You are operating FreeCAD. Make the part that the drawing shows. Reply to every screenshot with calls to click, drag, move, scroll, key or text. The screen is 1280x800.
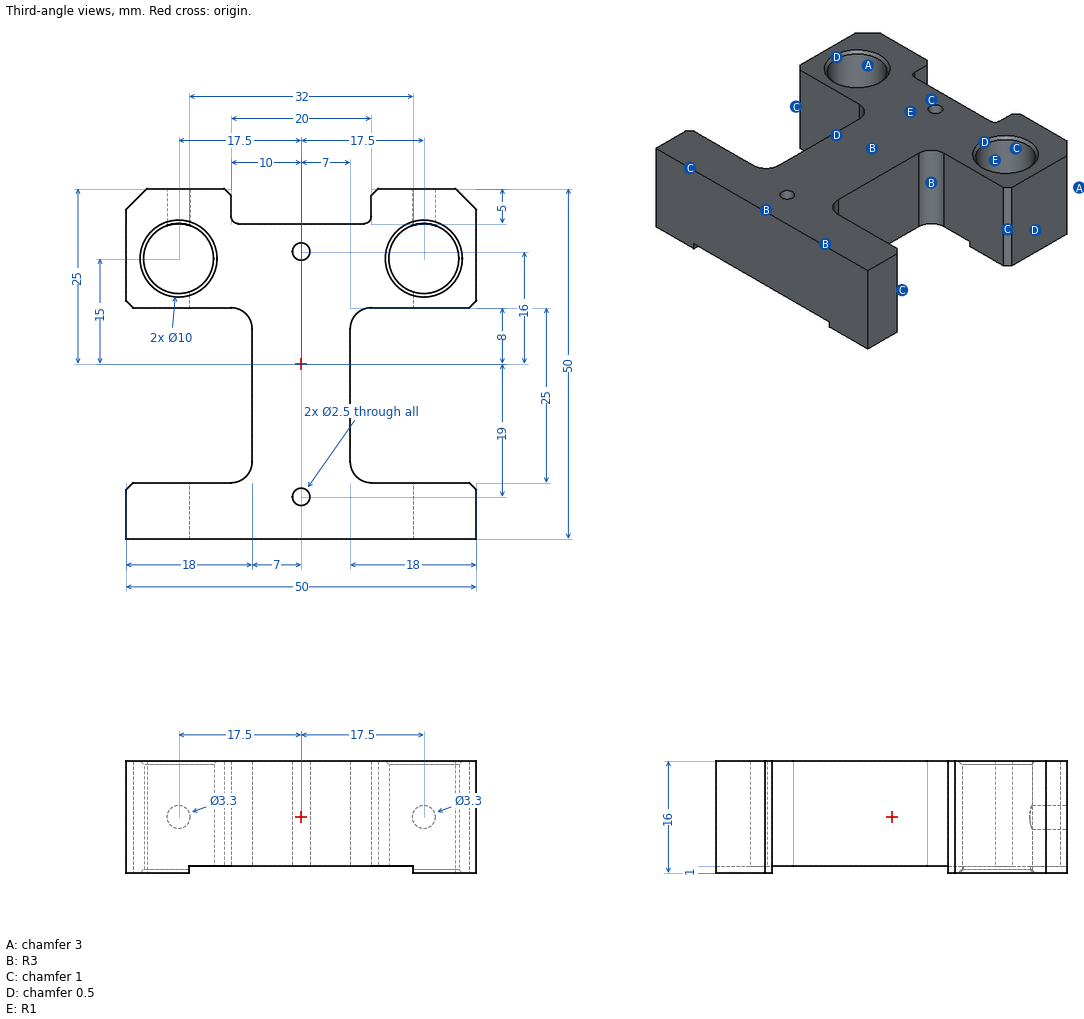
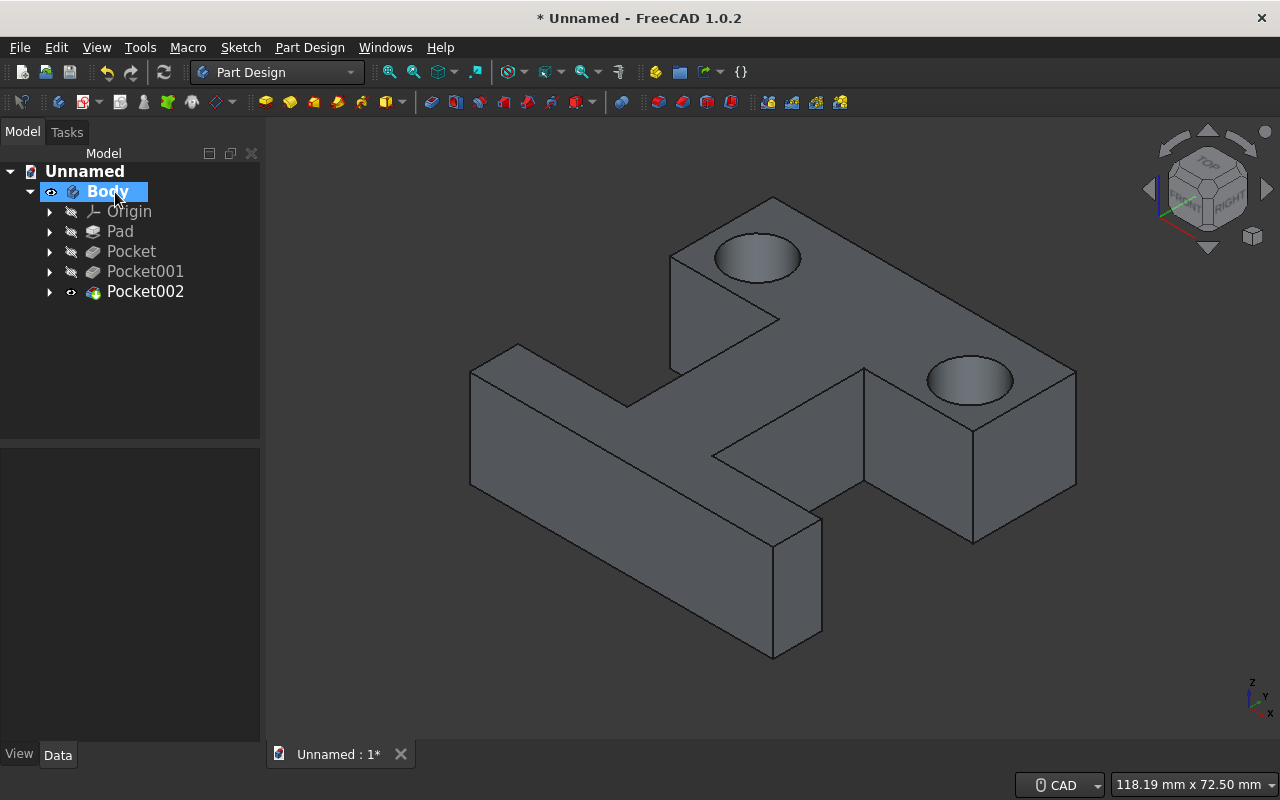
click(860, 321)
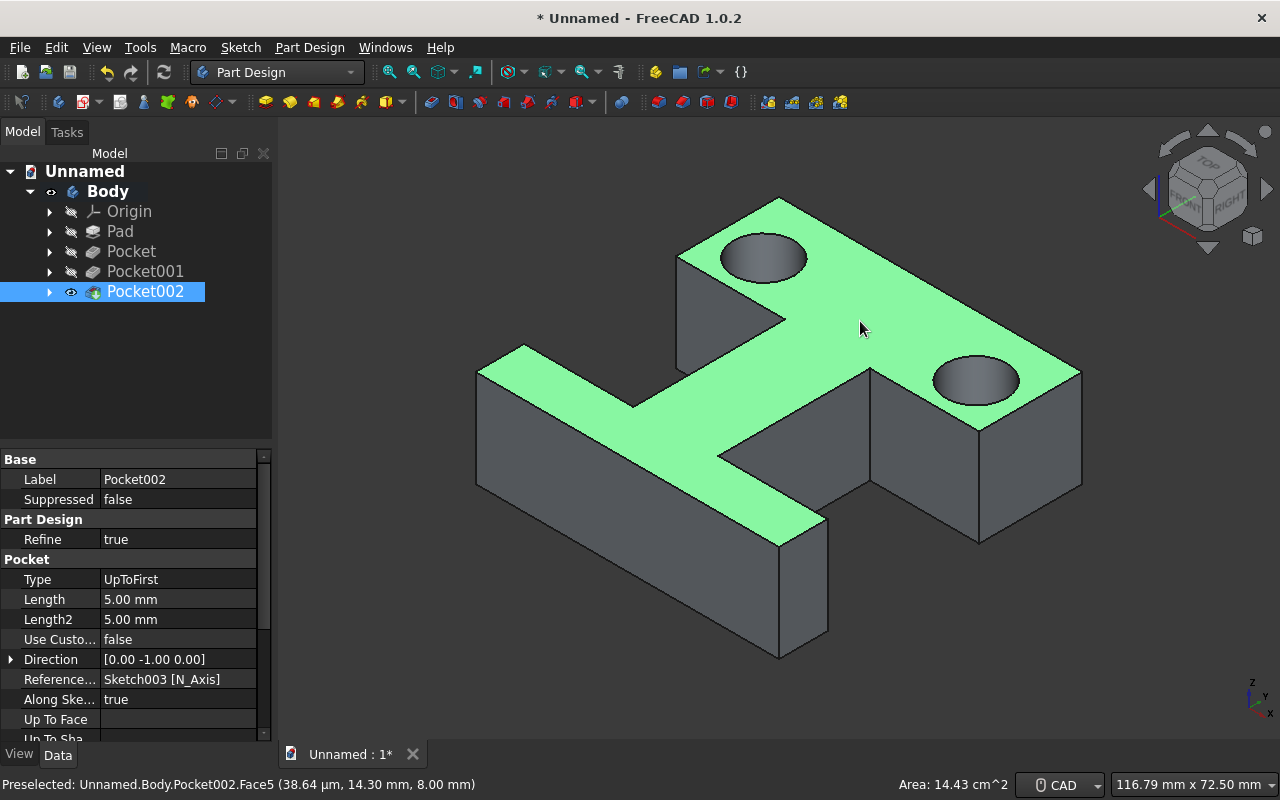
click(84, 102)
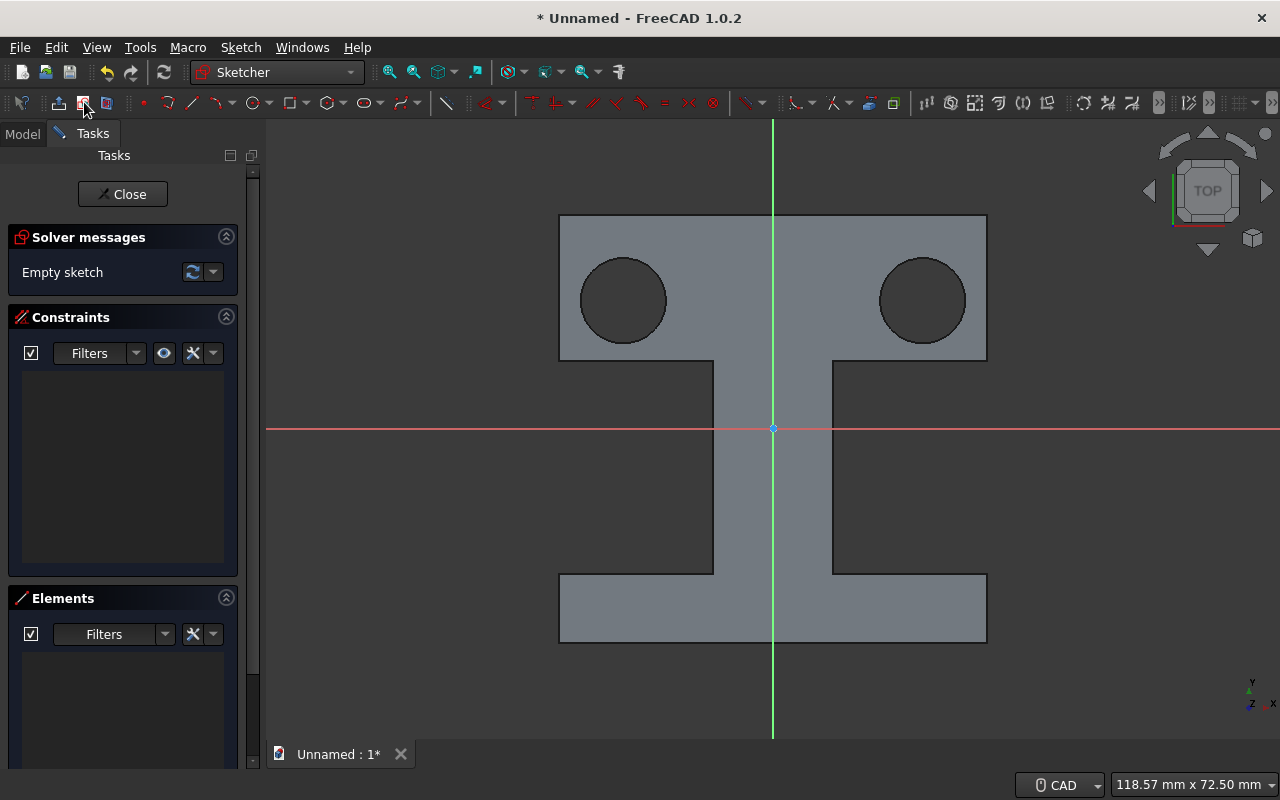
key(g)
key(c)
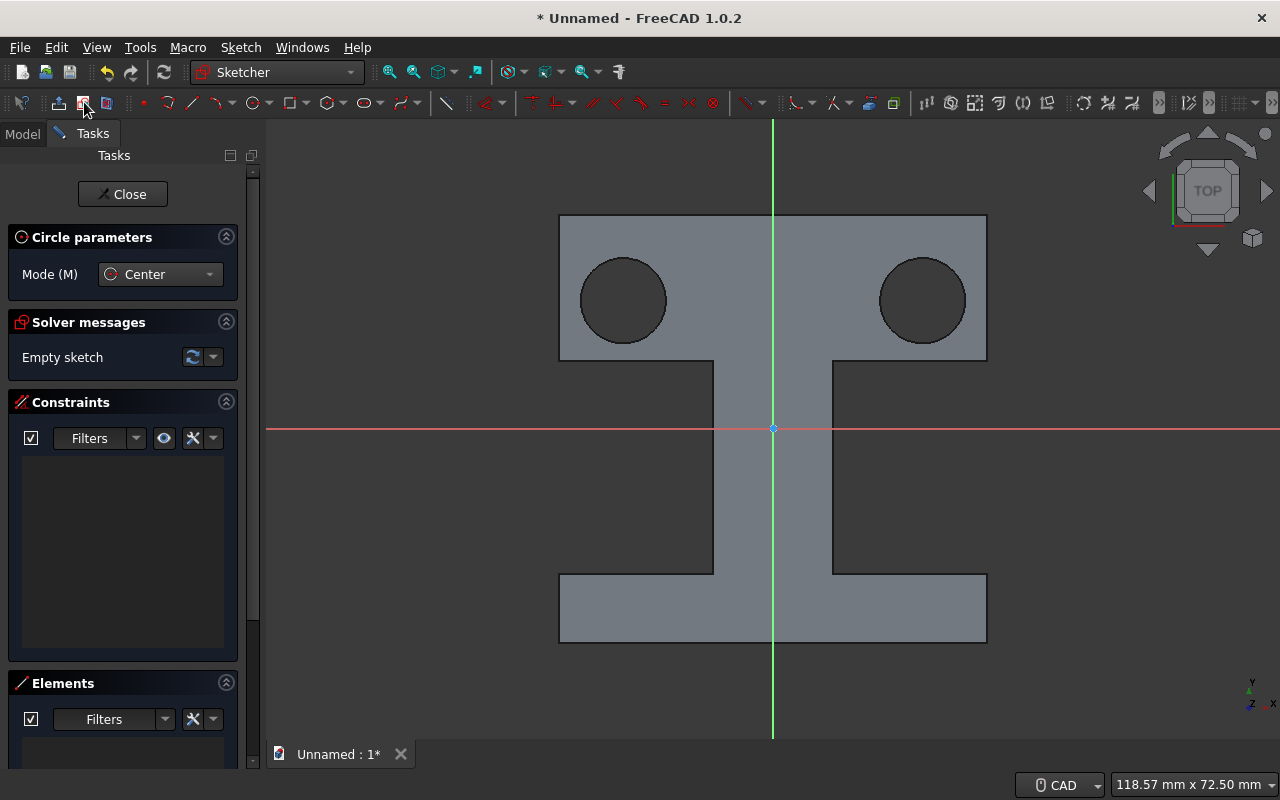
scroll(773, 591, up, 4)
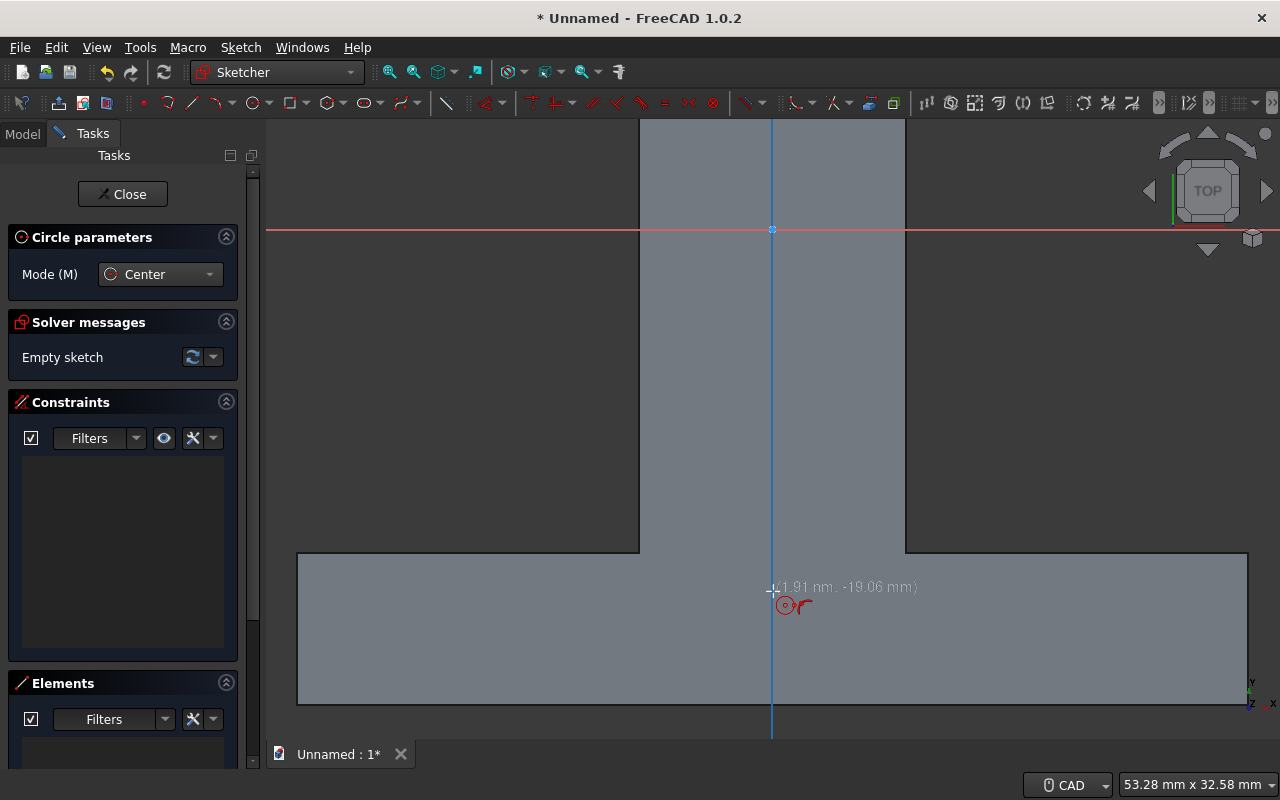
click(772, 591)
move(789, 574)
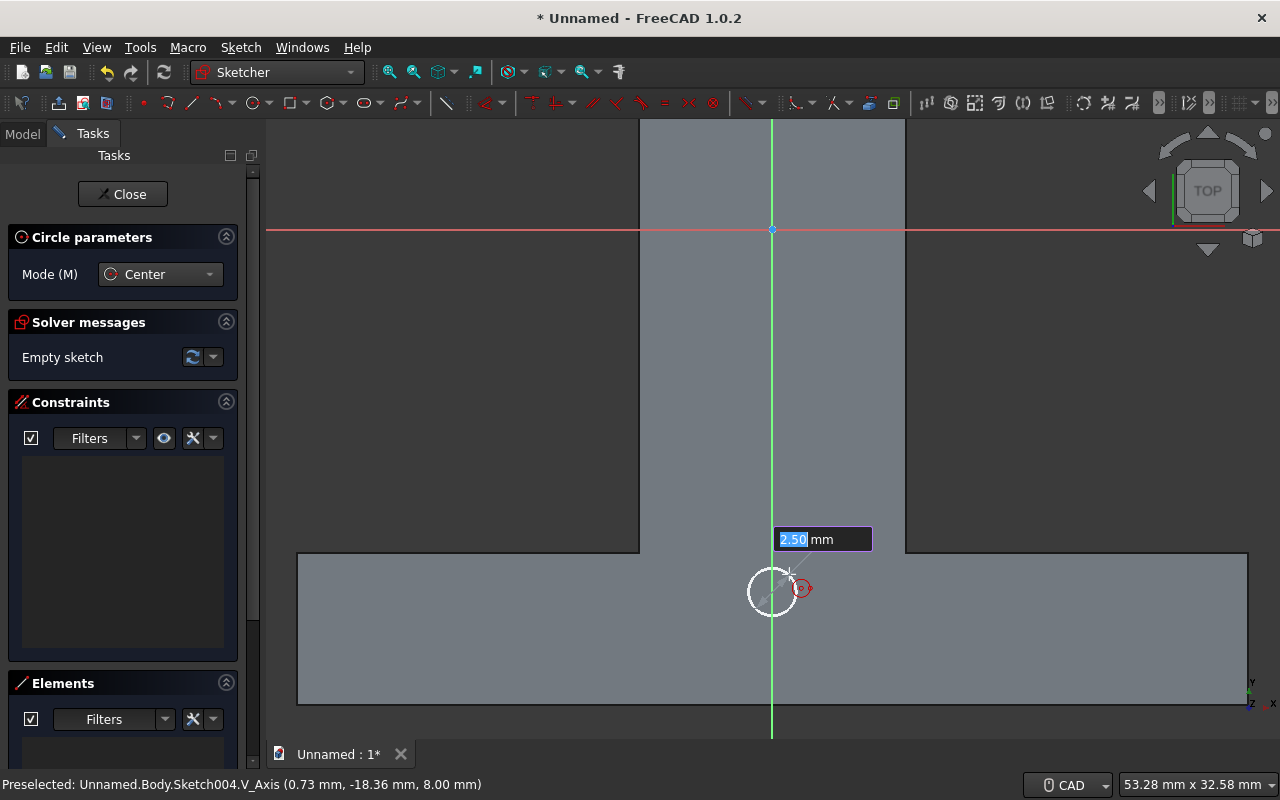
text(2.5)
key(Return)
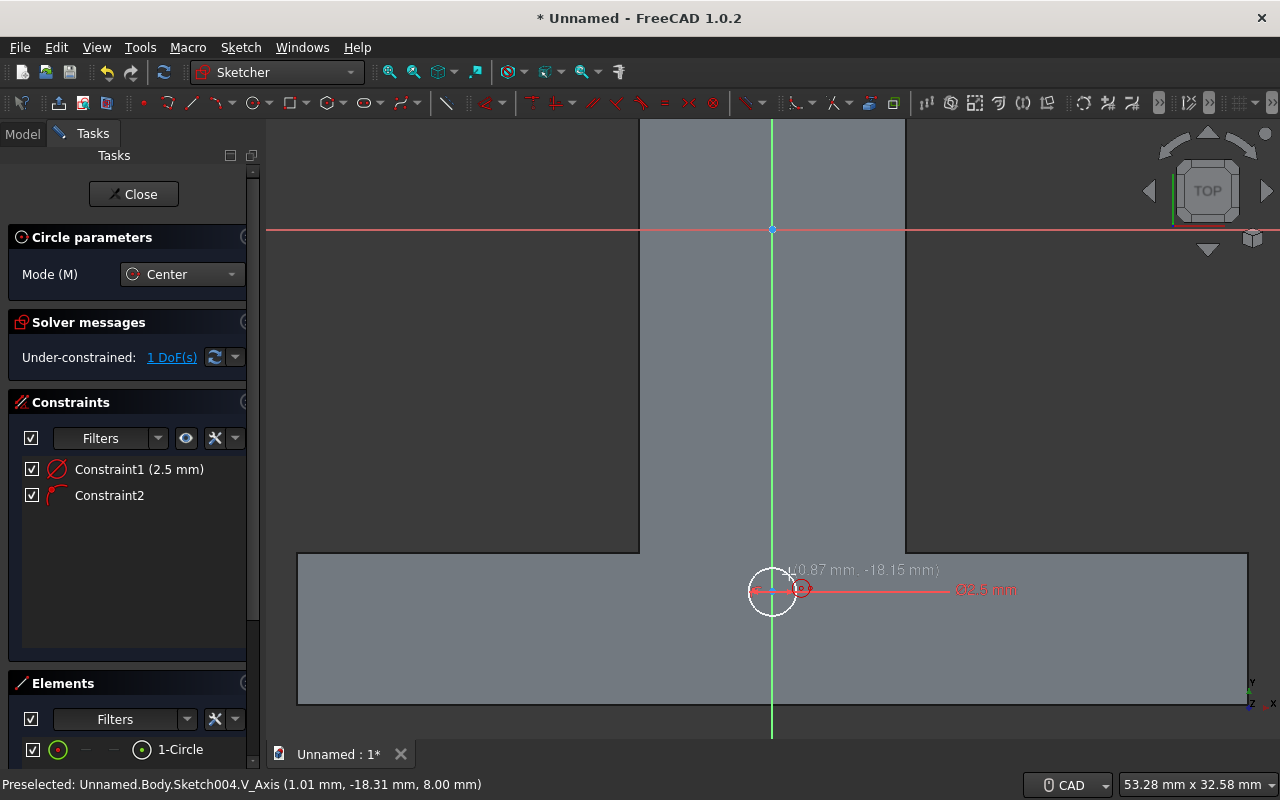
scroll(622, 637, down, 3)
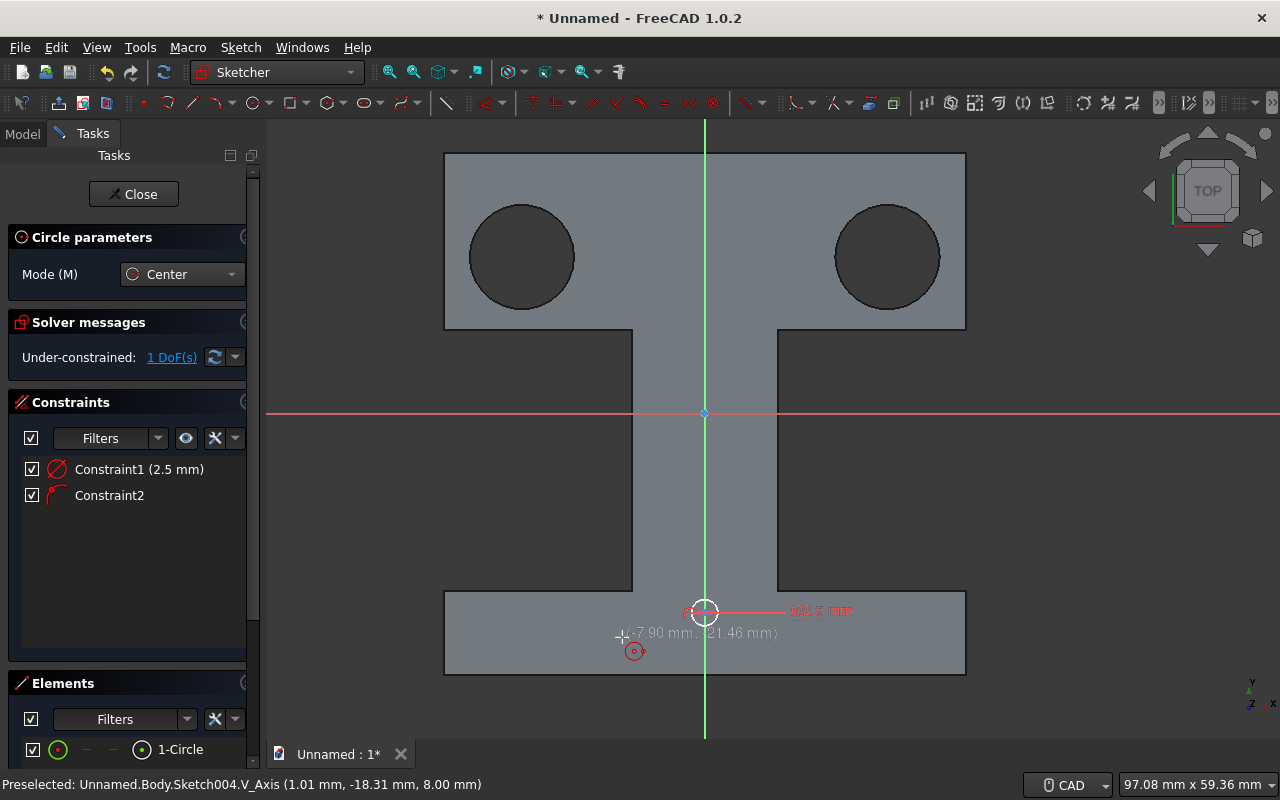
scroll(705, 247, up, 3)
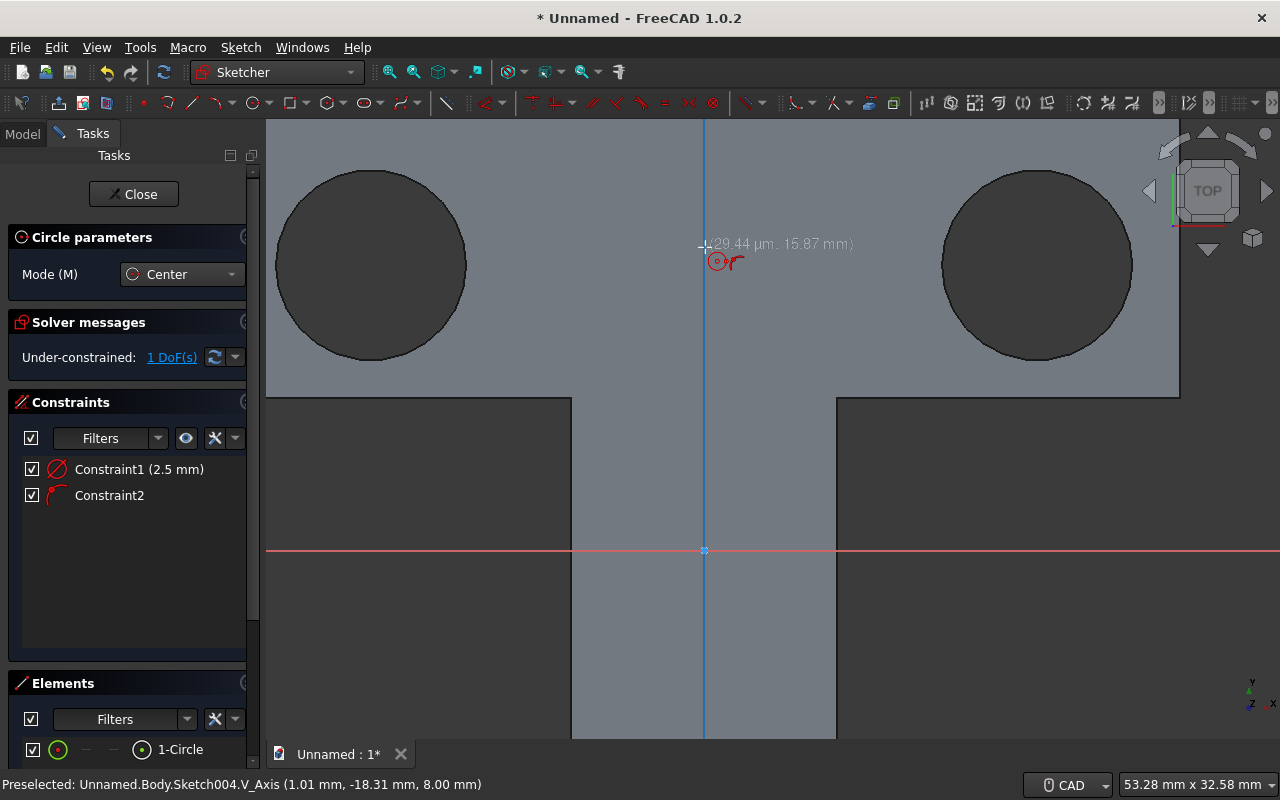
click(704, 246)
move(721, 229)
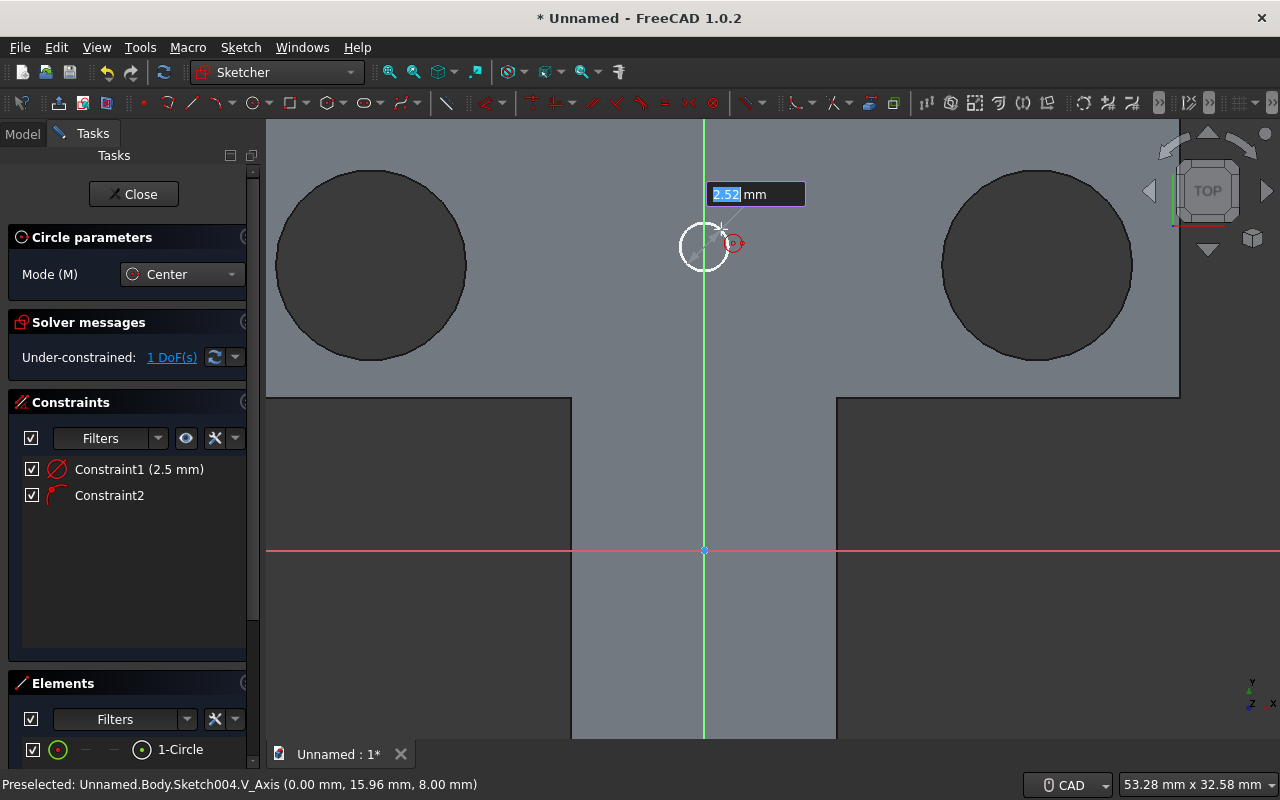
text(2.5)
key(Return)
key(Escape)